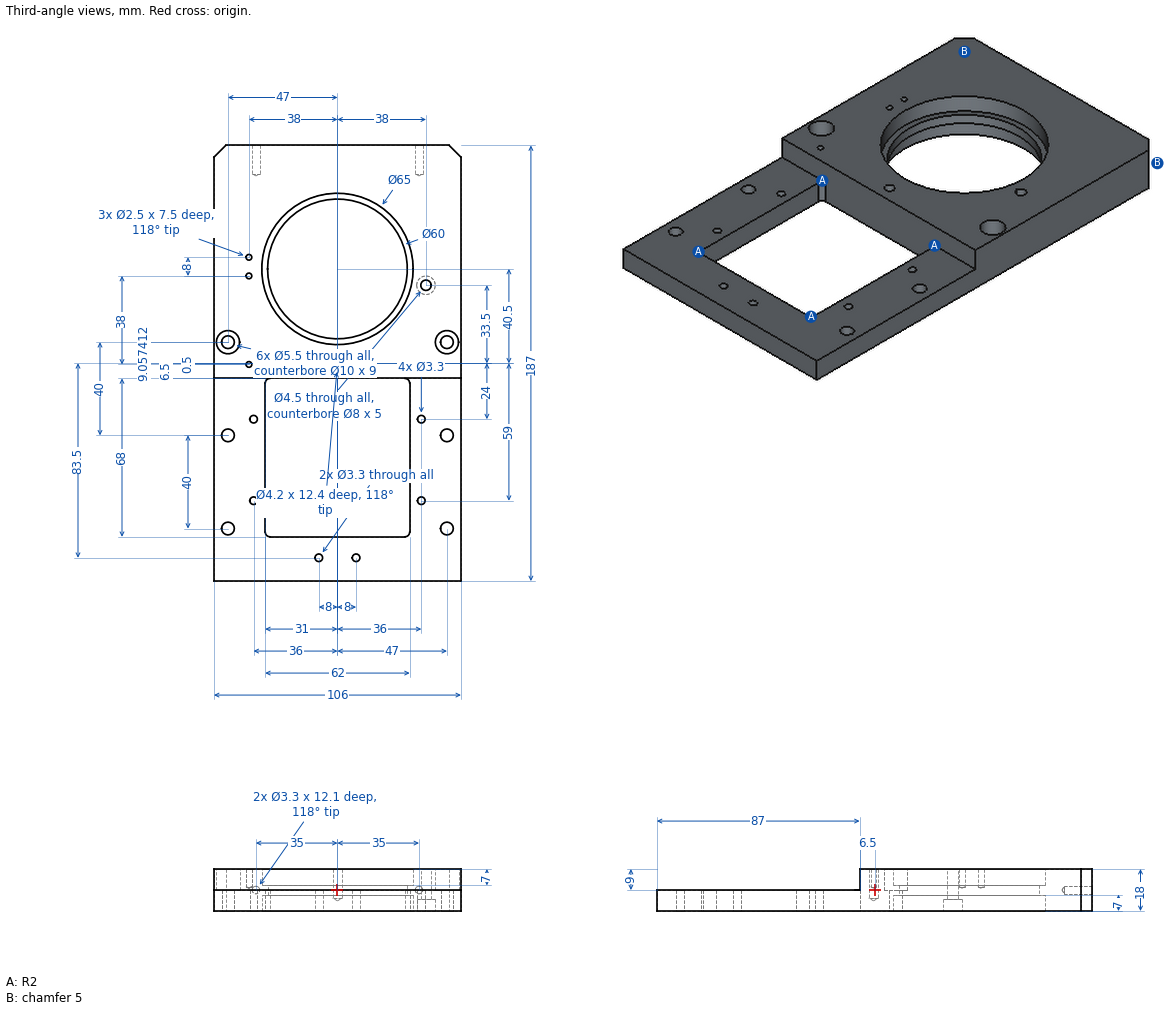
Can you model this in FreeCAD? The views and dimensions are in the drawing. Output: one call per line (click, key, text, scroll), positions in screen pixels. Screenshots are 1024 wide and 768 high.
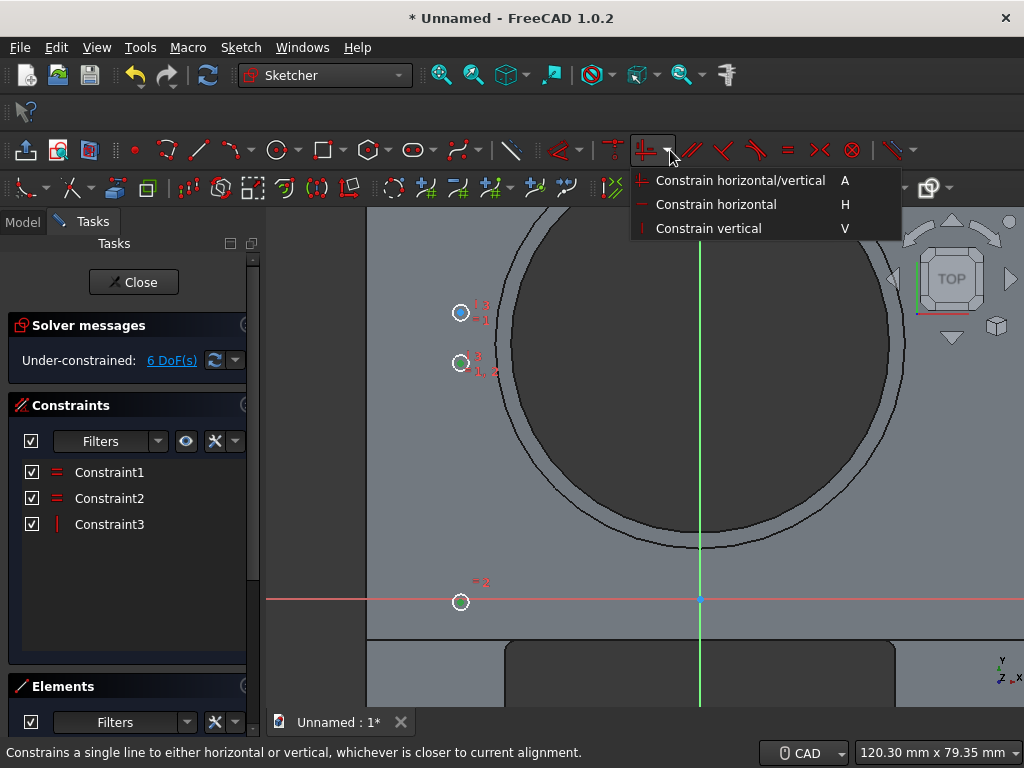
click(766, 228)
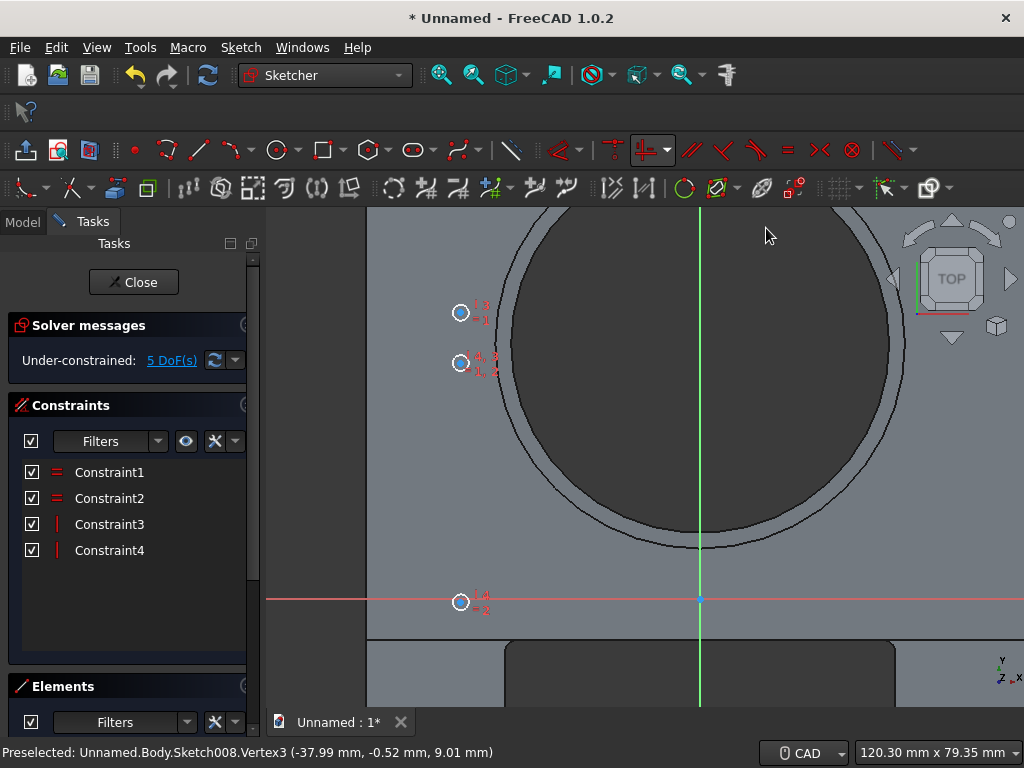
click(558, 150)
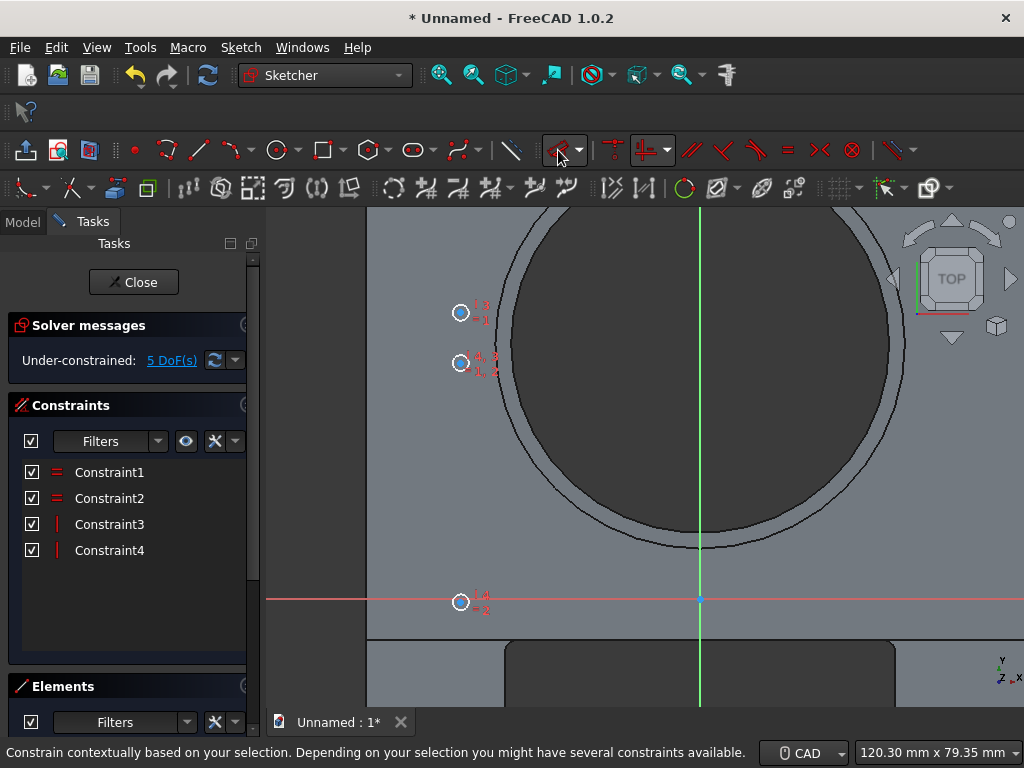
scroll(461, 305, up, 5)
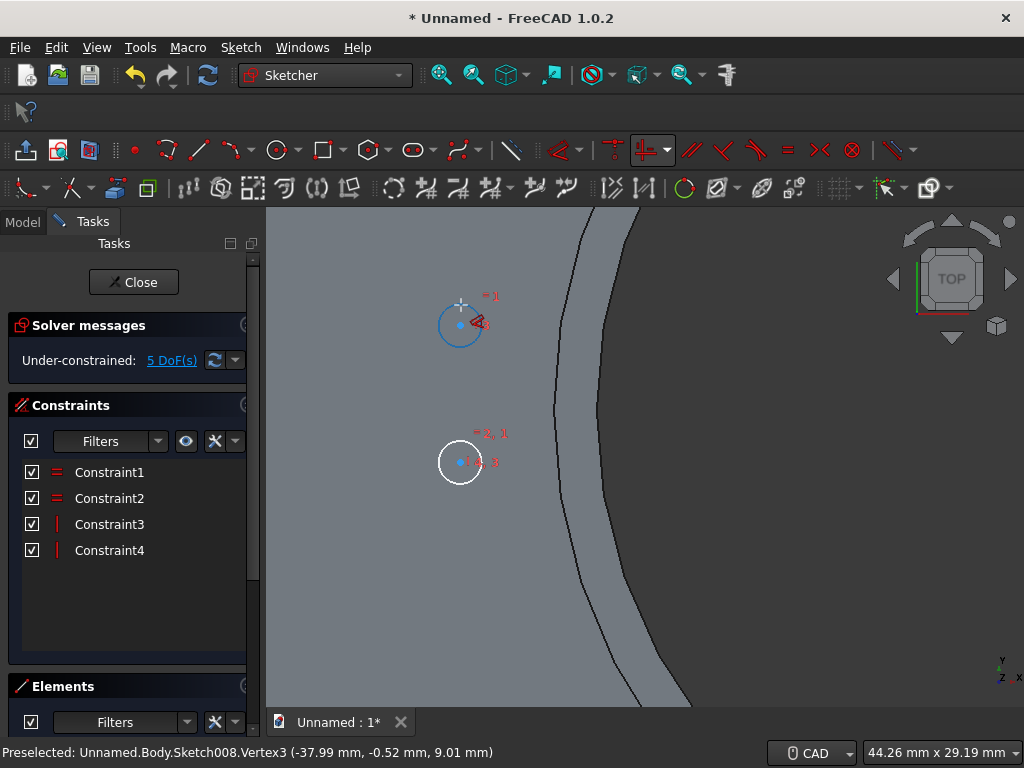
click(461, 304)
click(462, 272)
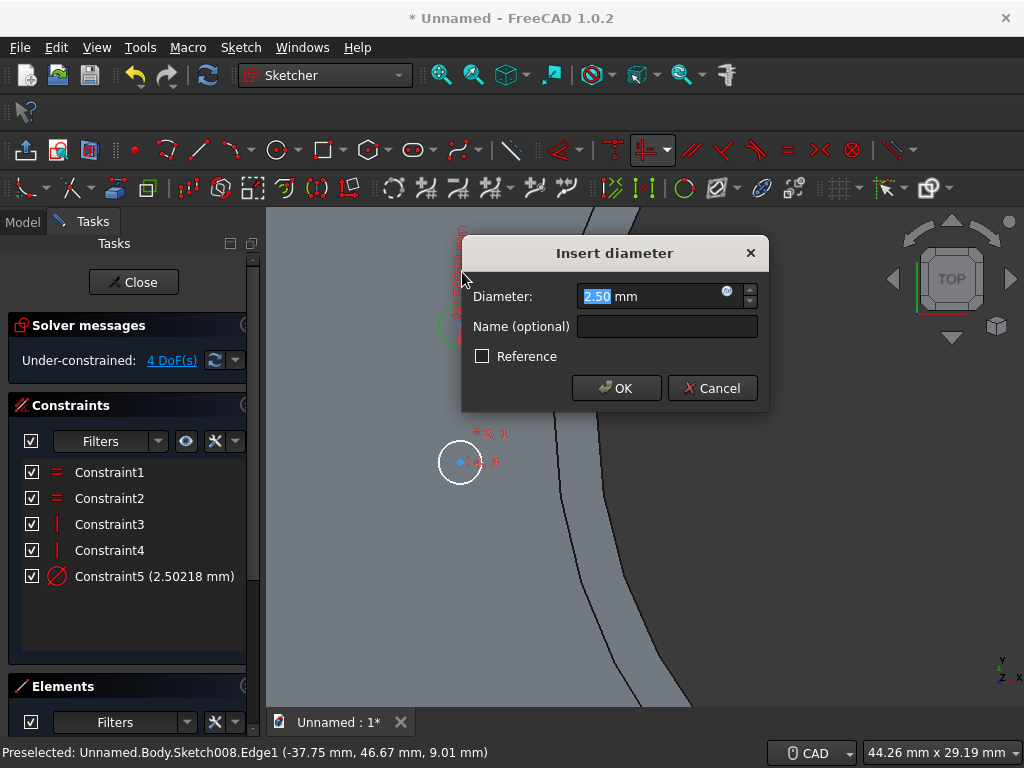
text(2.5)
key(Return)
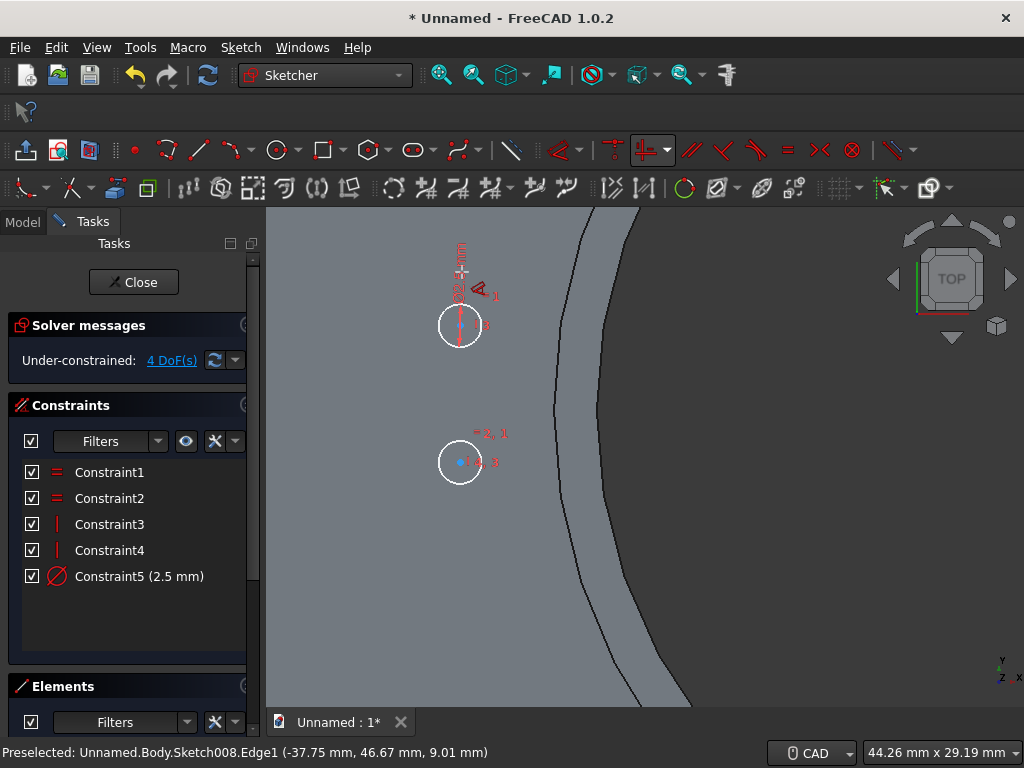
click(460, 326)
click(660, 292)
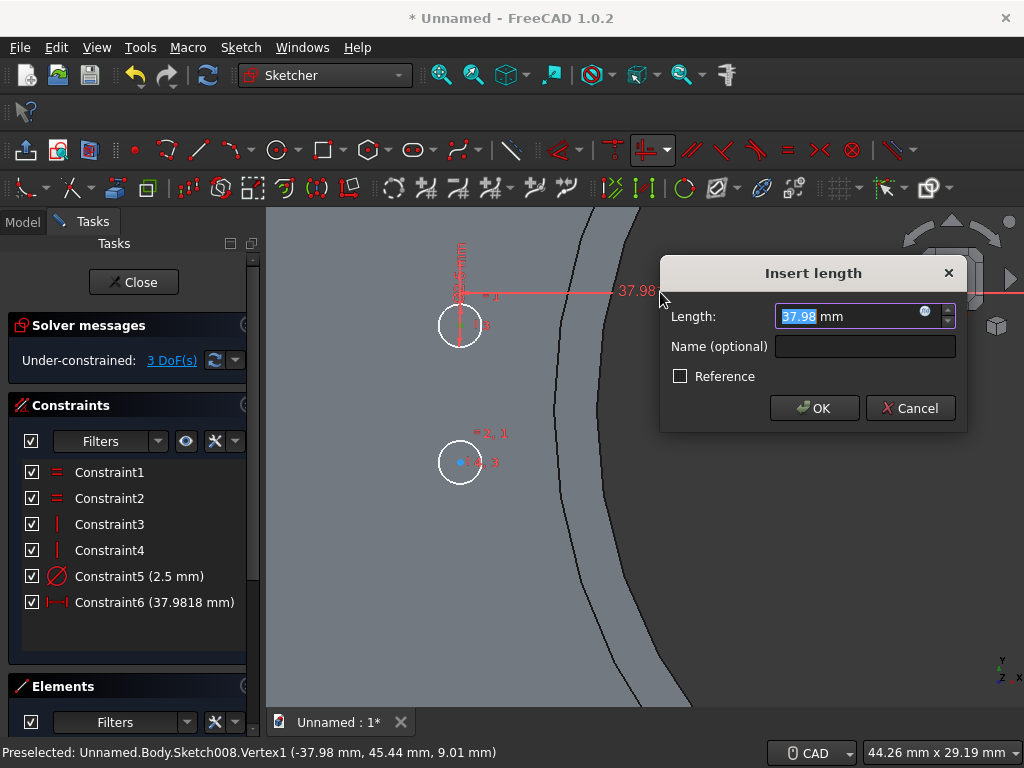
text(38)
key(Return)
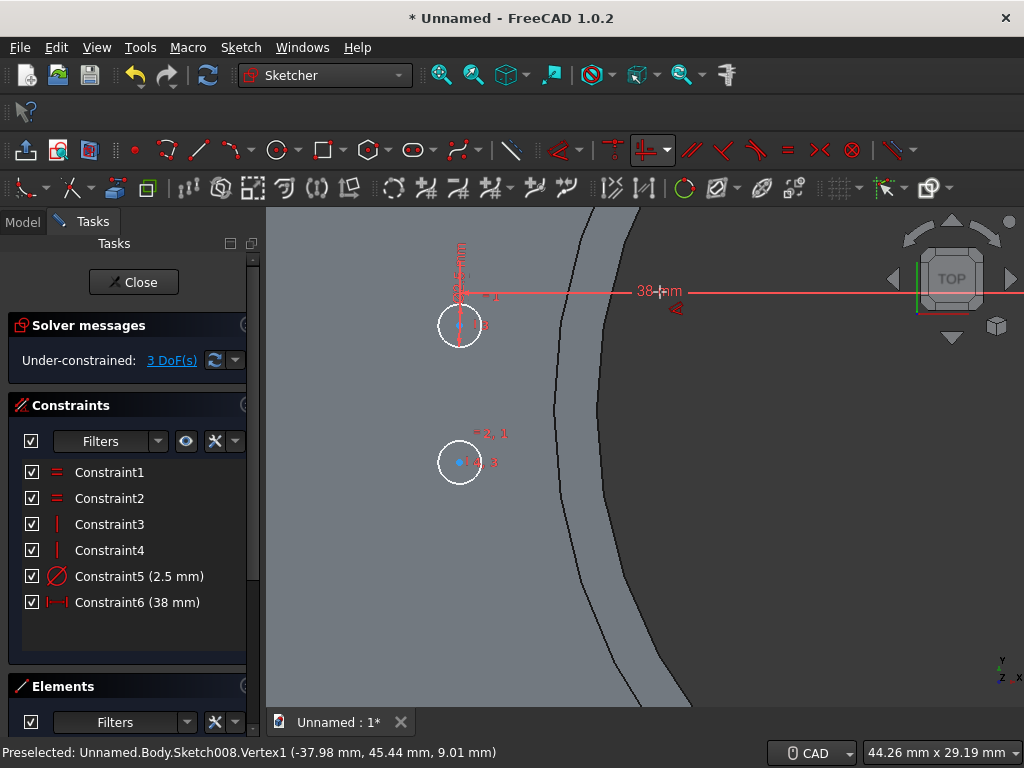
click(460, 326)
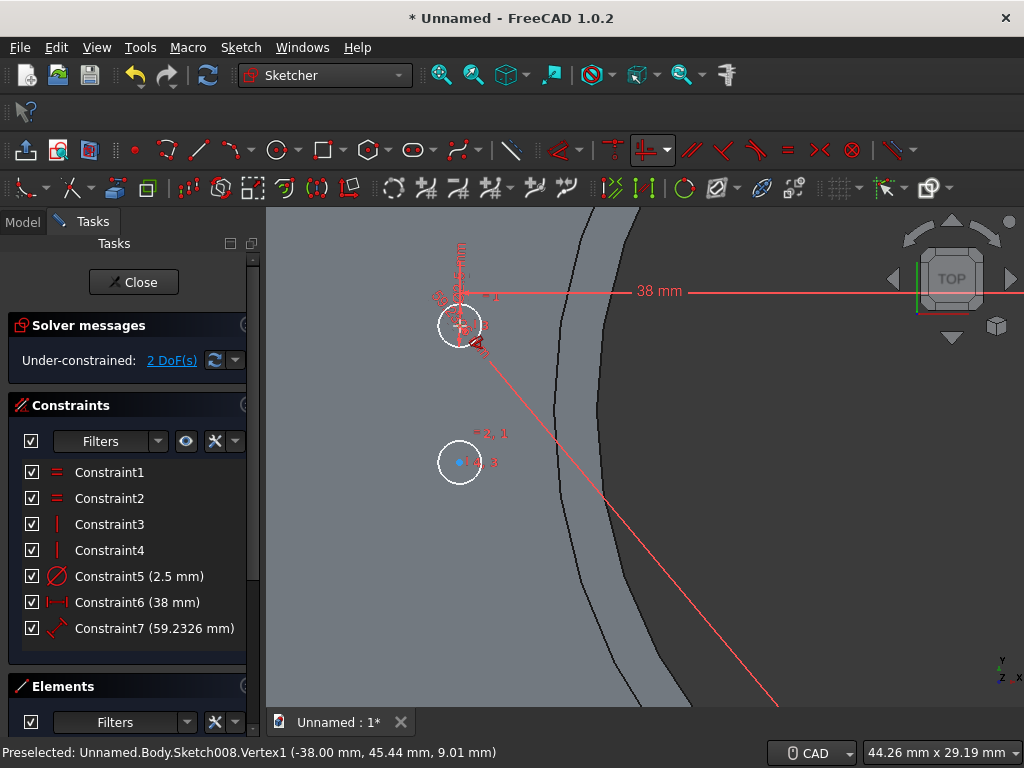
click(460, 462)
click(426, 394)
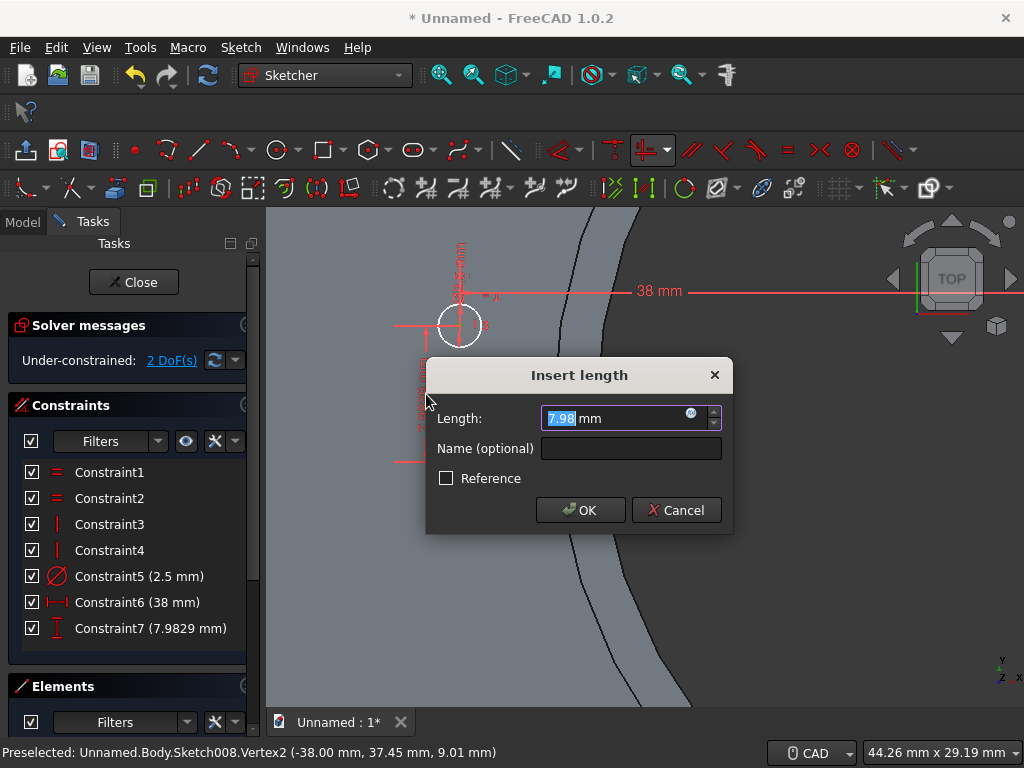
text(8)
key(Return)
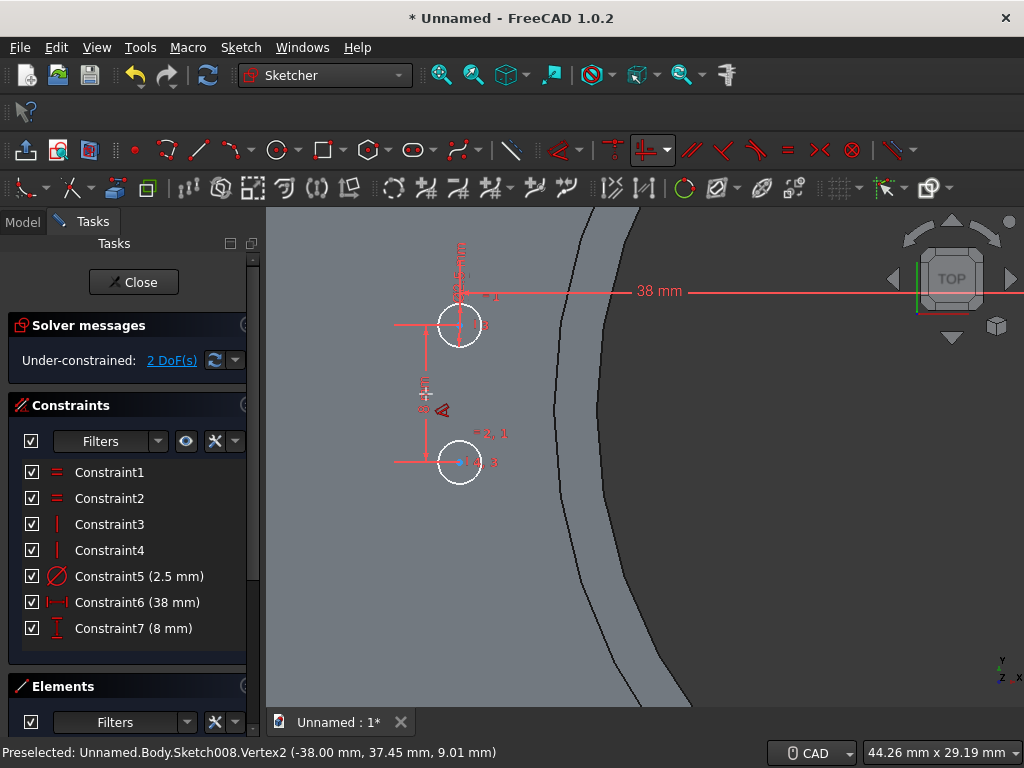
scroll(461, 305, down, 5)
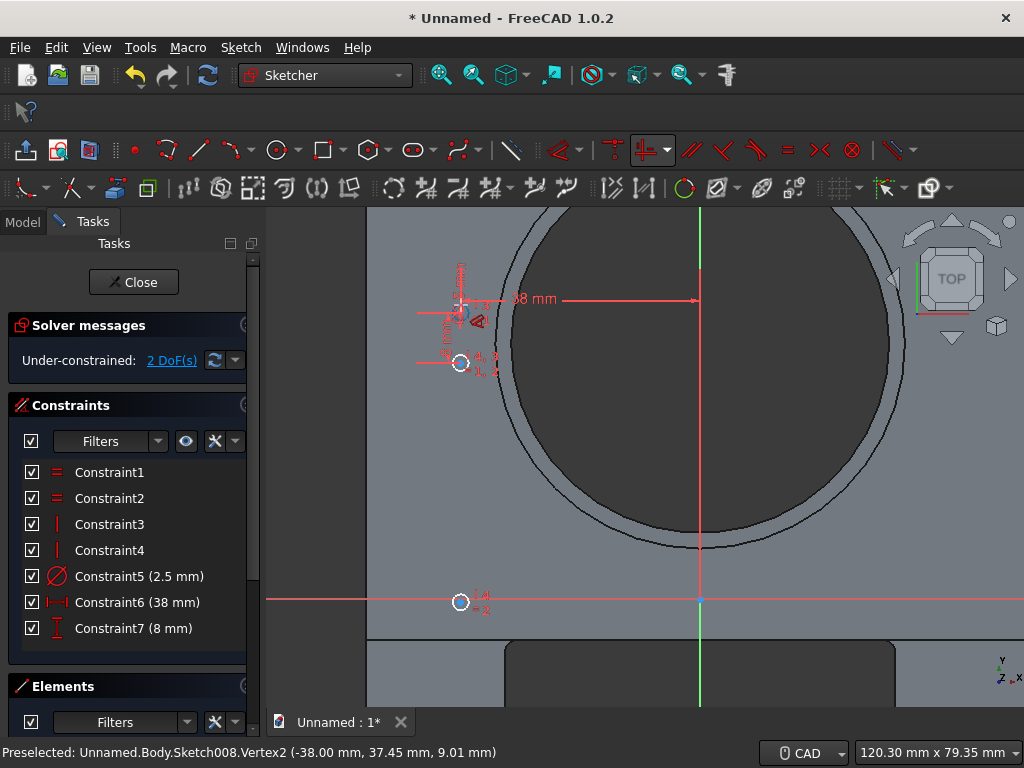
scroll(461, 602, up, 13)